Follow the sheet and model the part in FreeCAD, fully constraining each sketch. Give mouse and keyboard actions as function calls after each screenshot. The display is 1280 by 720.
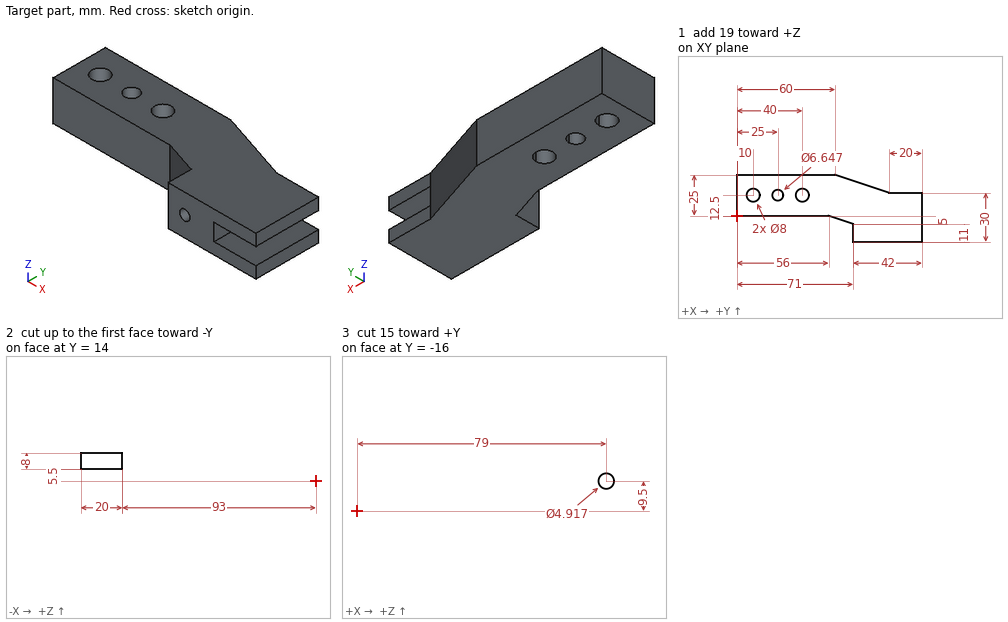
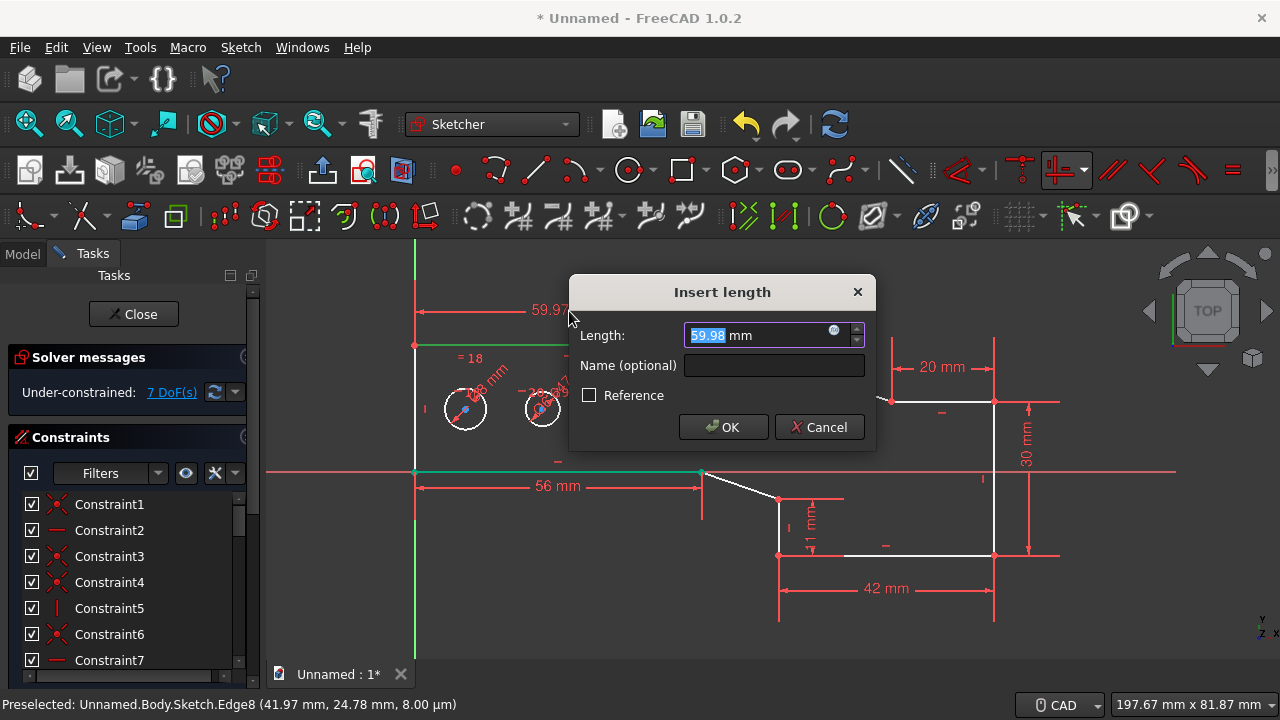
text(60)
key(Return)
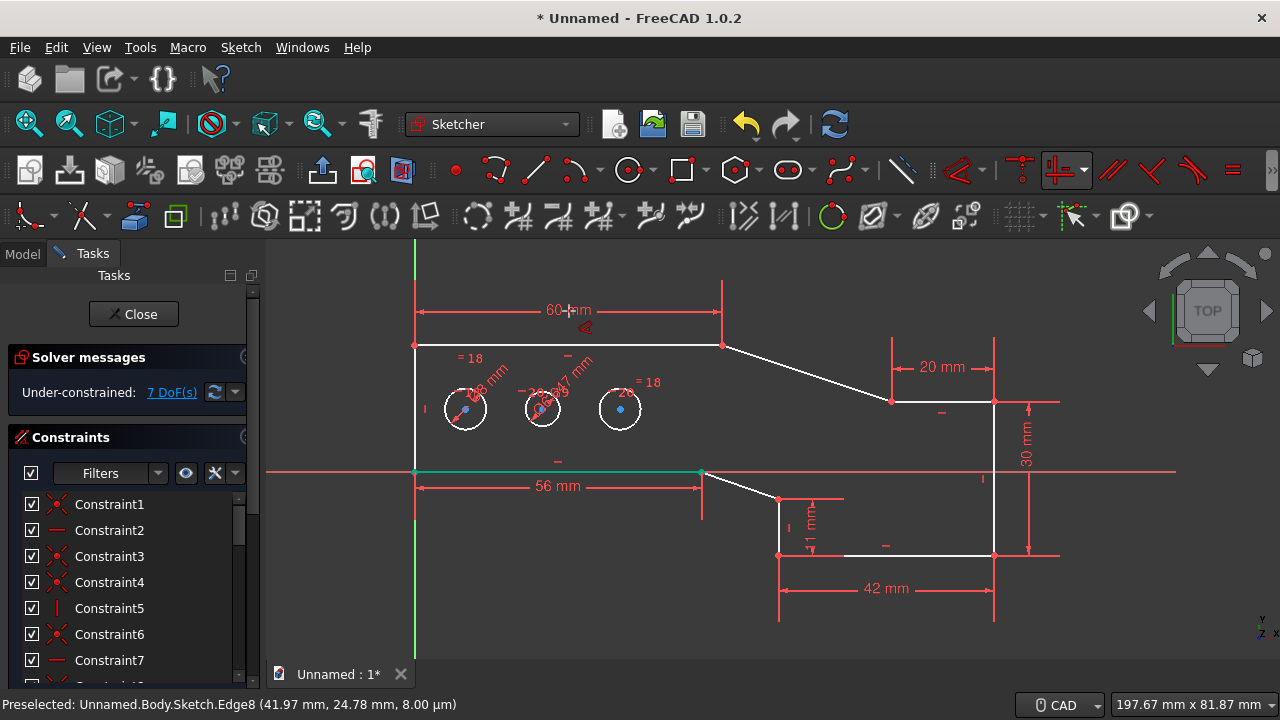
click(415, 384)
click(381, 409)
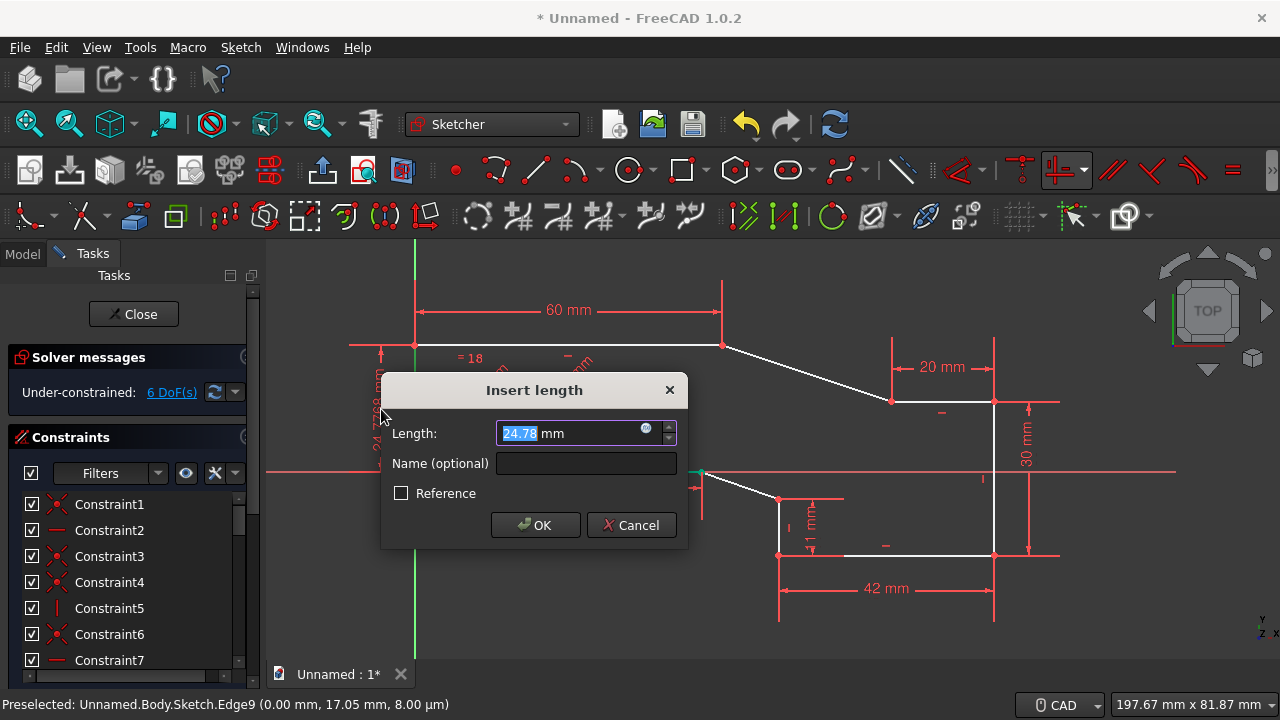
text(25)
key(Return)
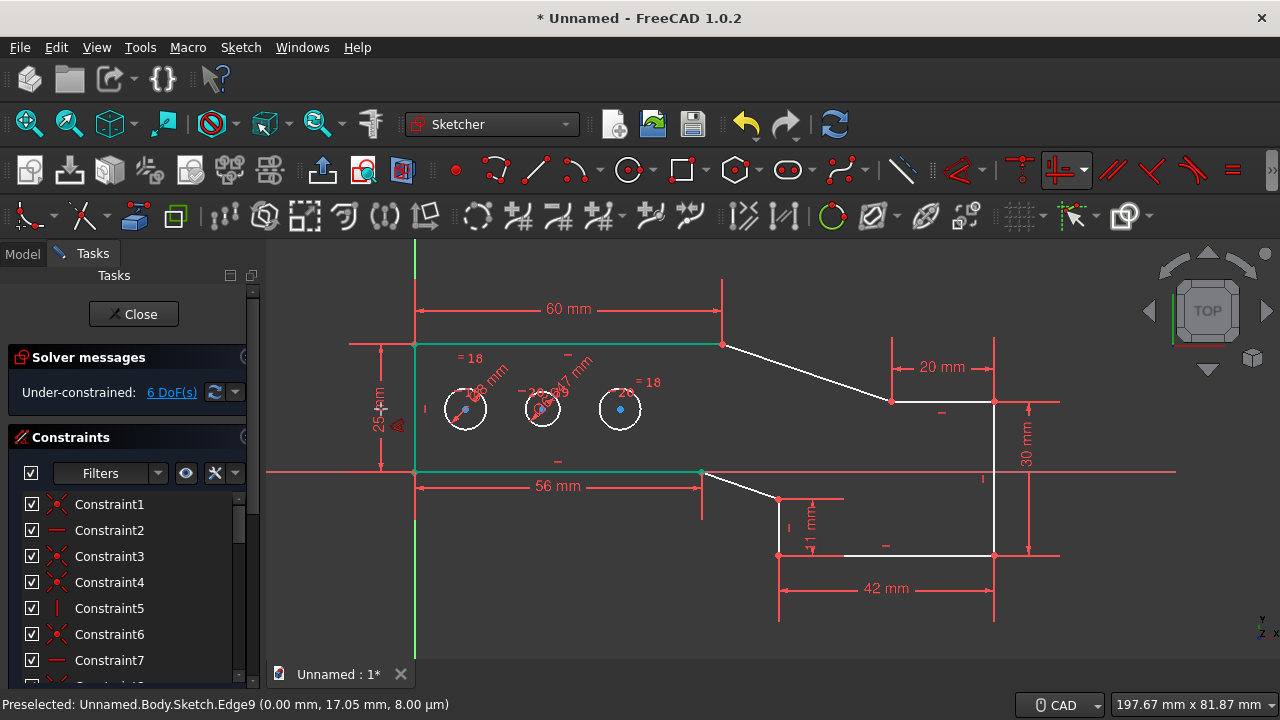
scroll(779, 499, up, 3)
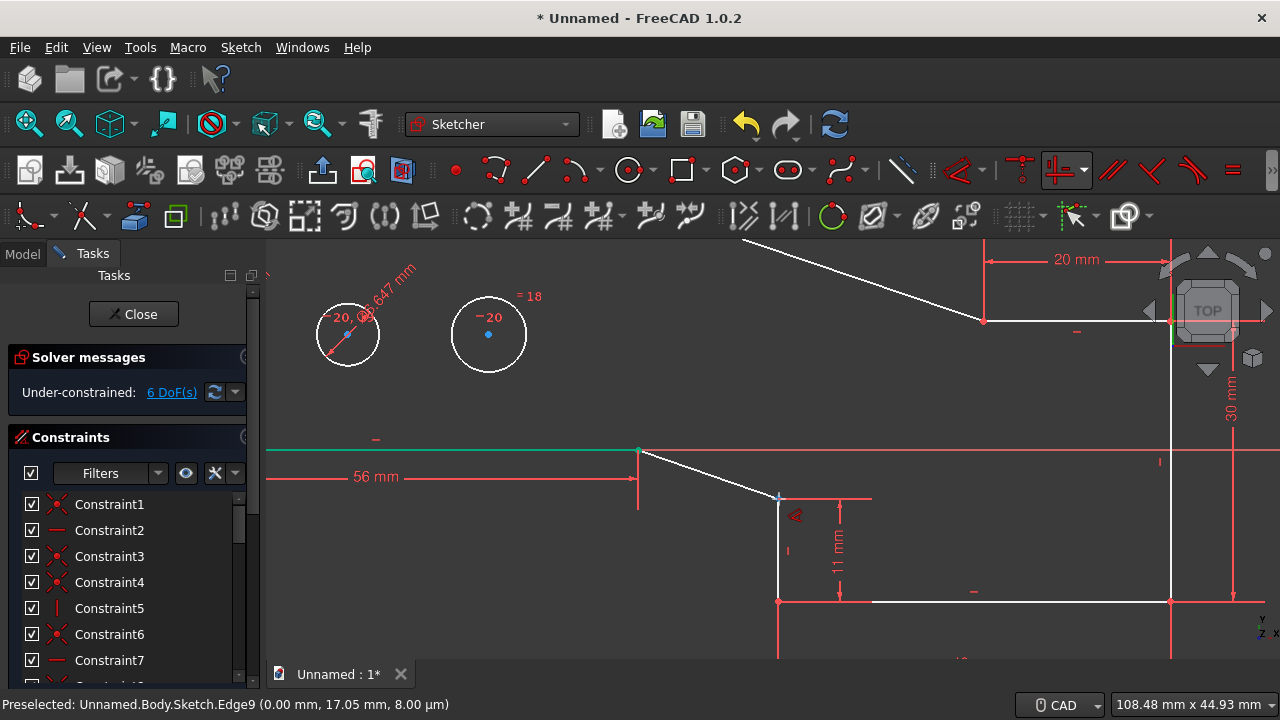
click(778, 499)
click(812, 475)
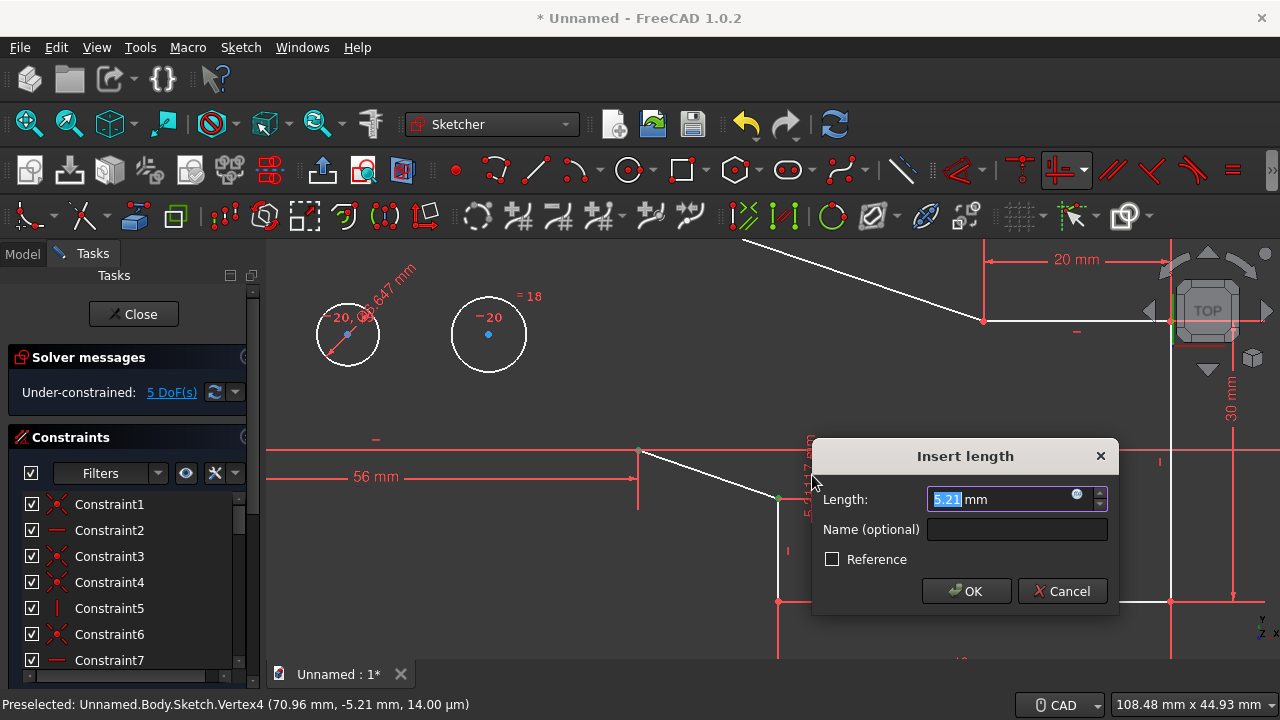
text(5)
key(Return)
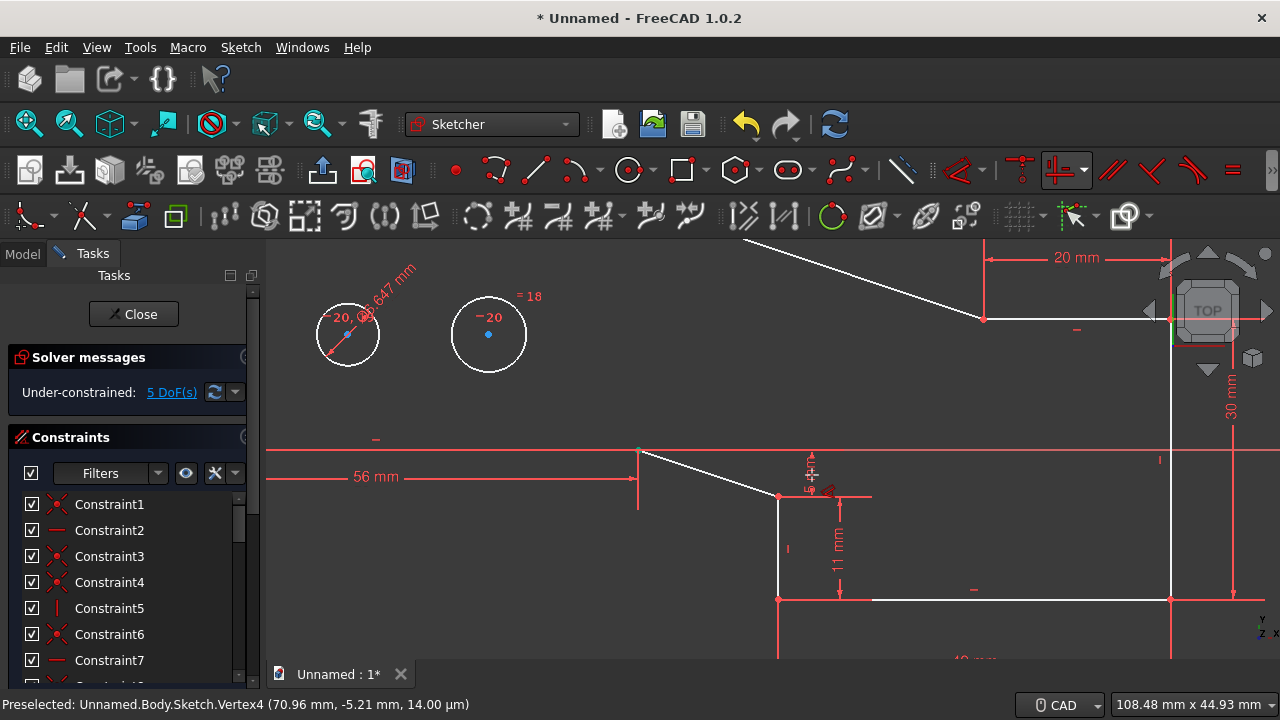
scroll(779, 499, down, 3)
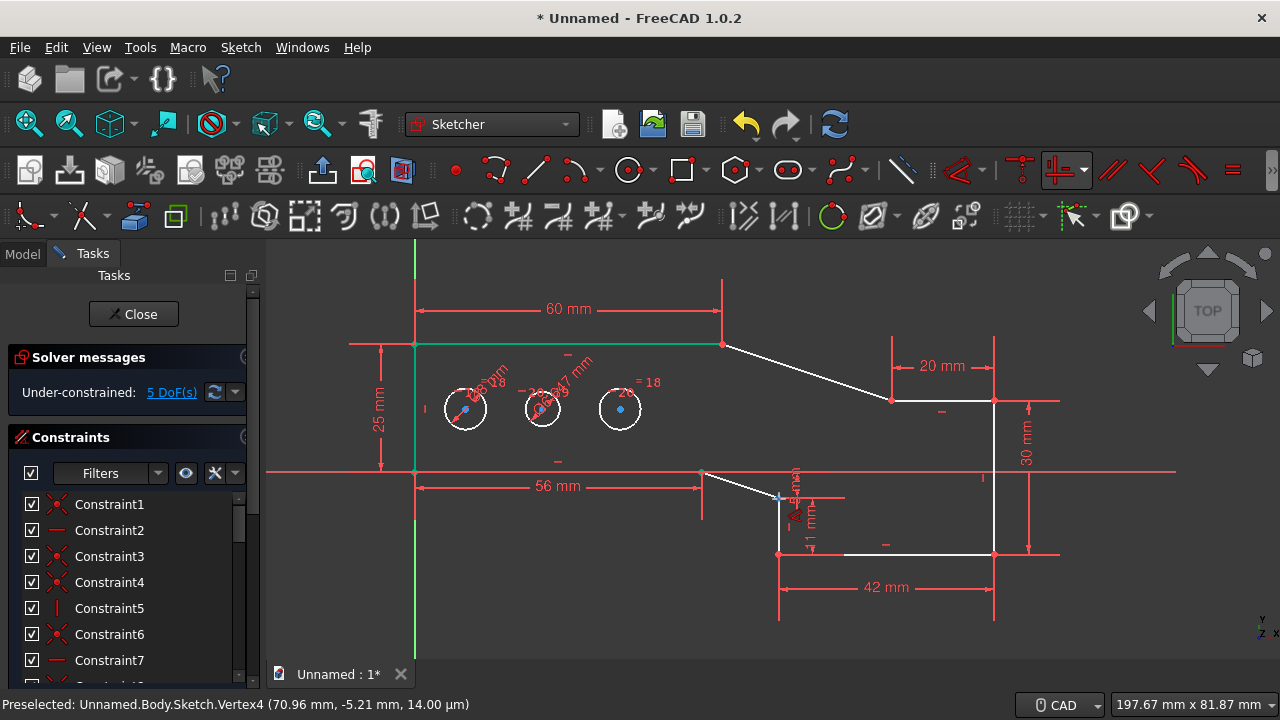
click(466, 409)
click(440, 506)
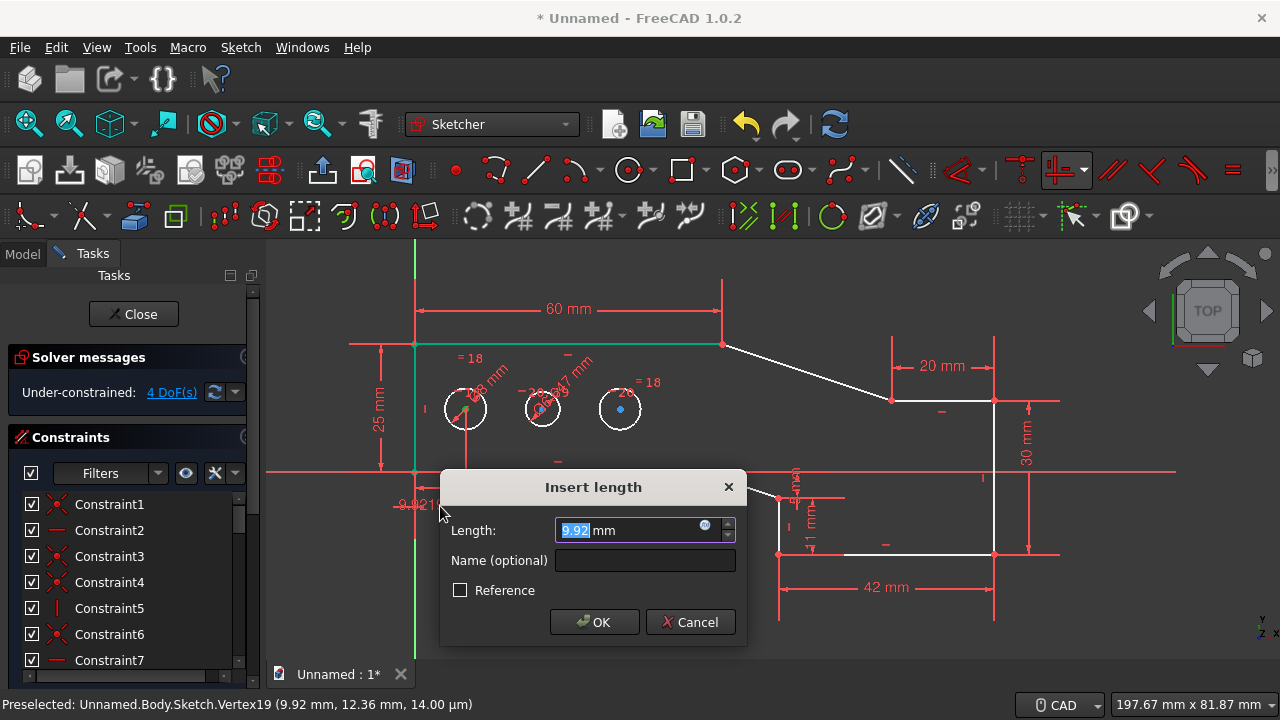
text(10)
key(Return)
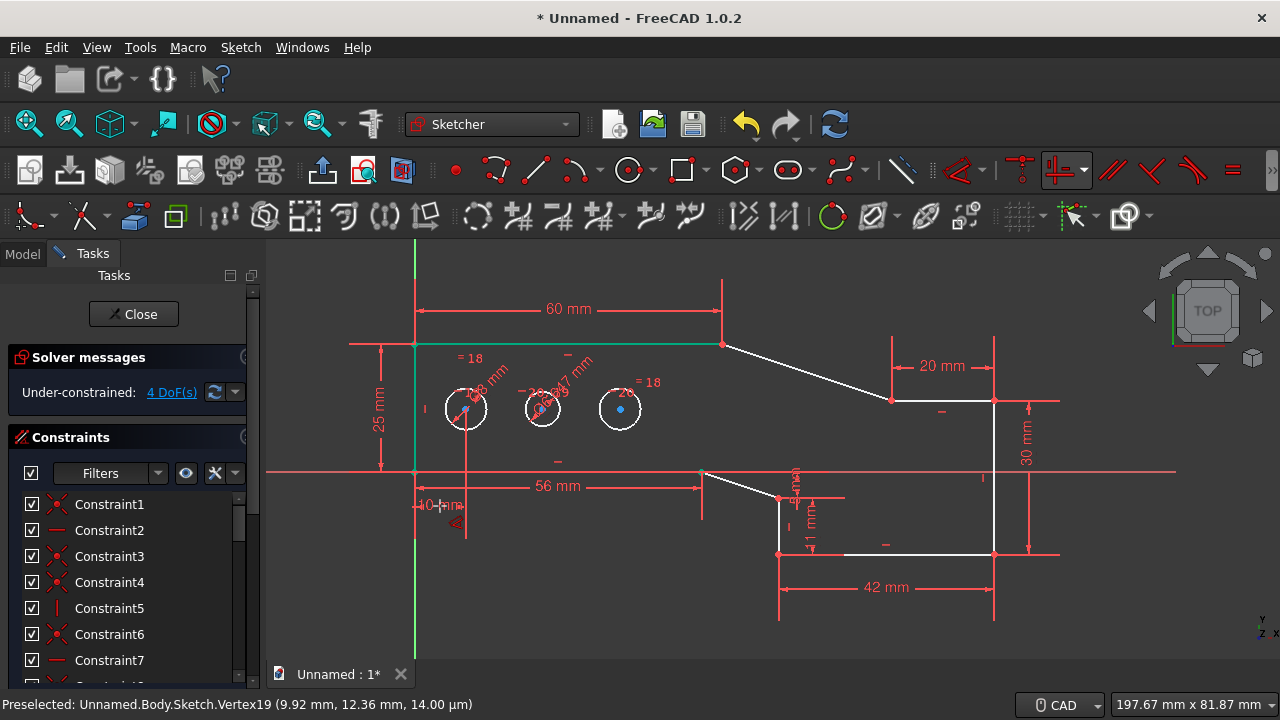
click(543, 409)
click(479, 530)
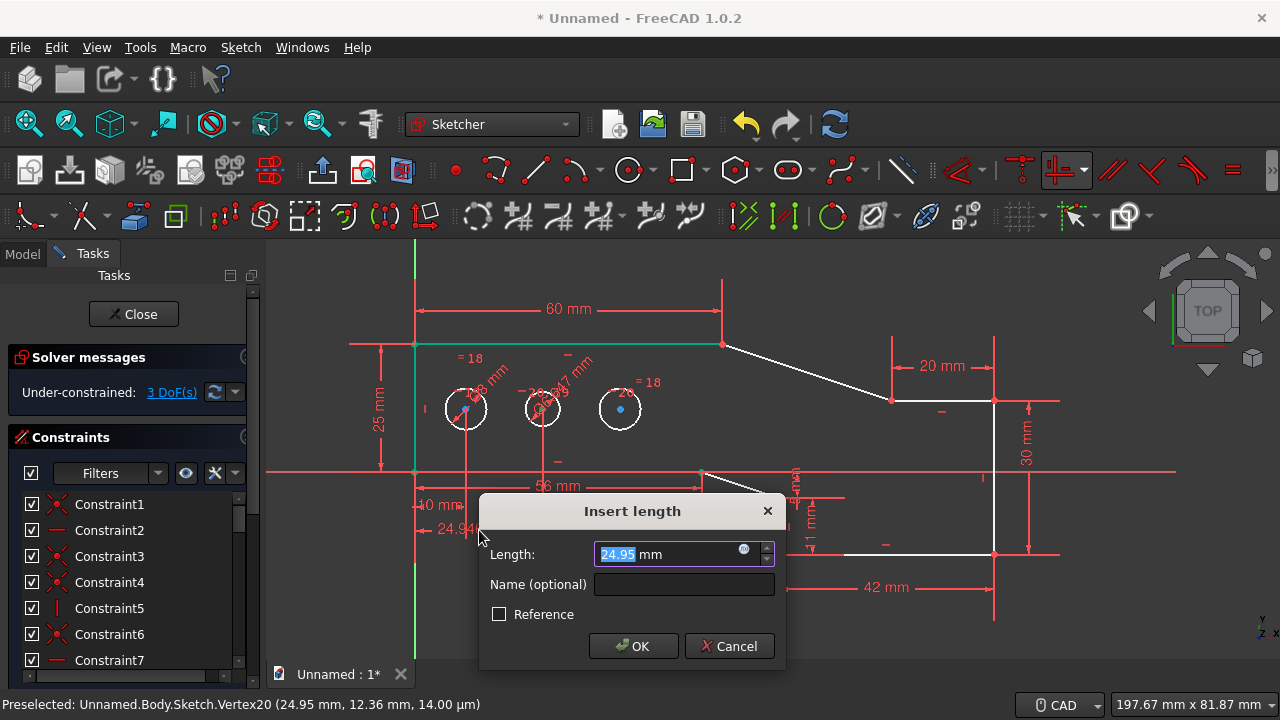
text(25)
key(Return)